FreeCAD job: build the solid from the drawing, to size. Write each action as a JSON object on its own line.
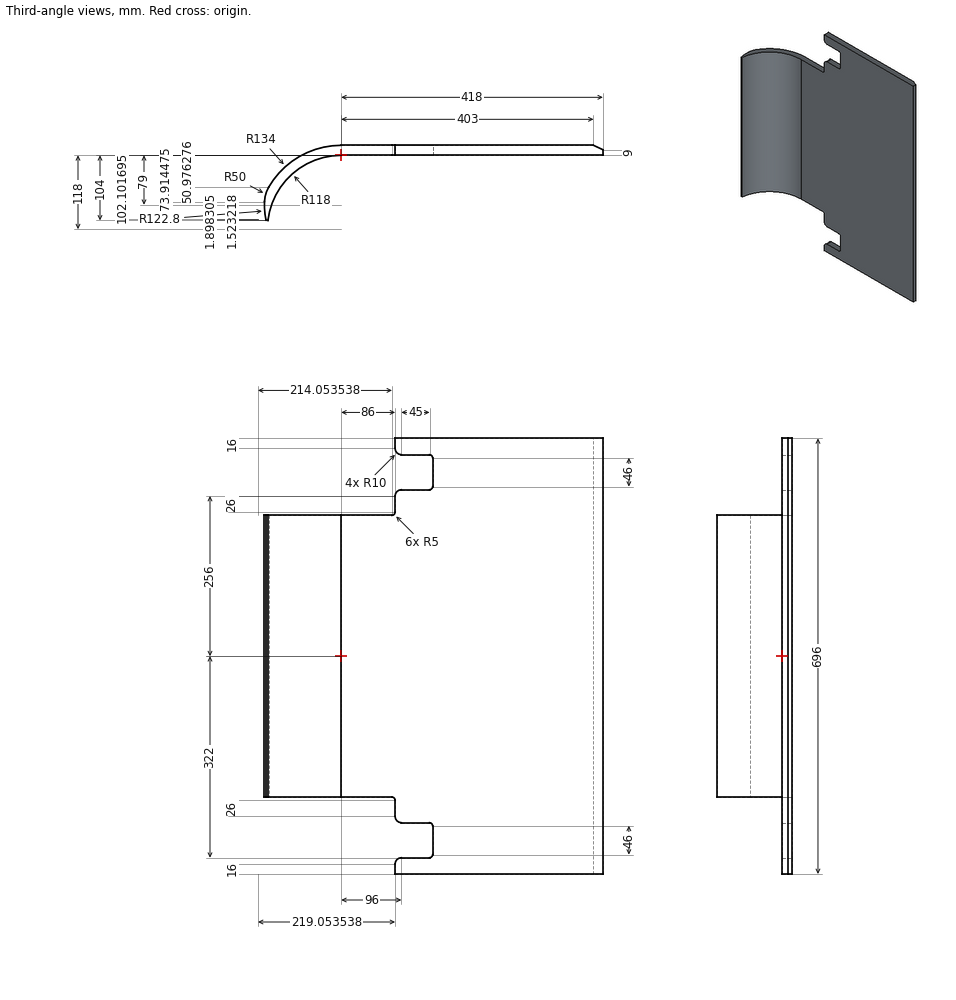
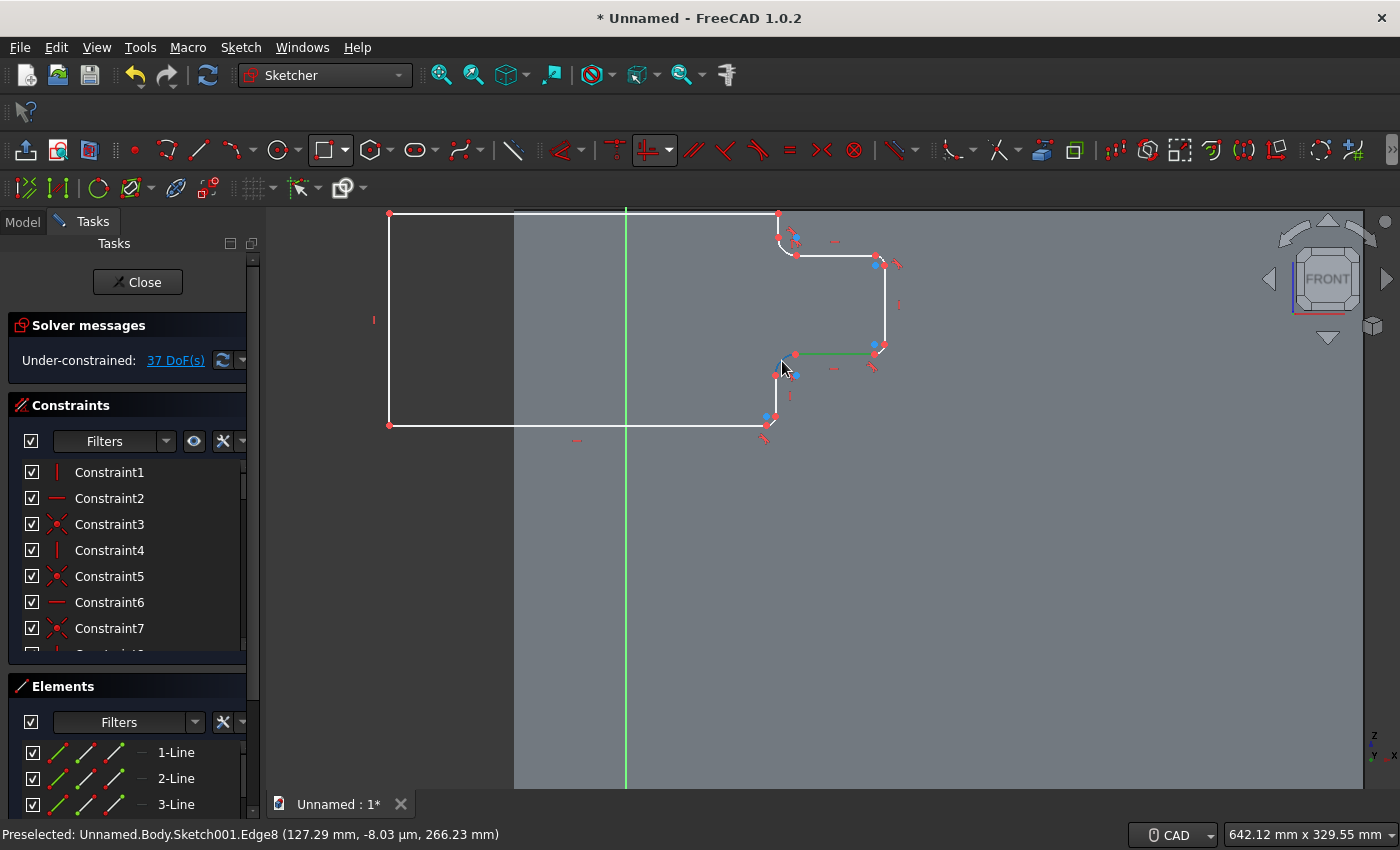
{"action": "left_click", "coordinate": [781, 361]}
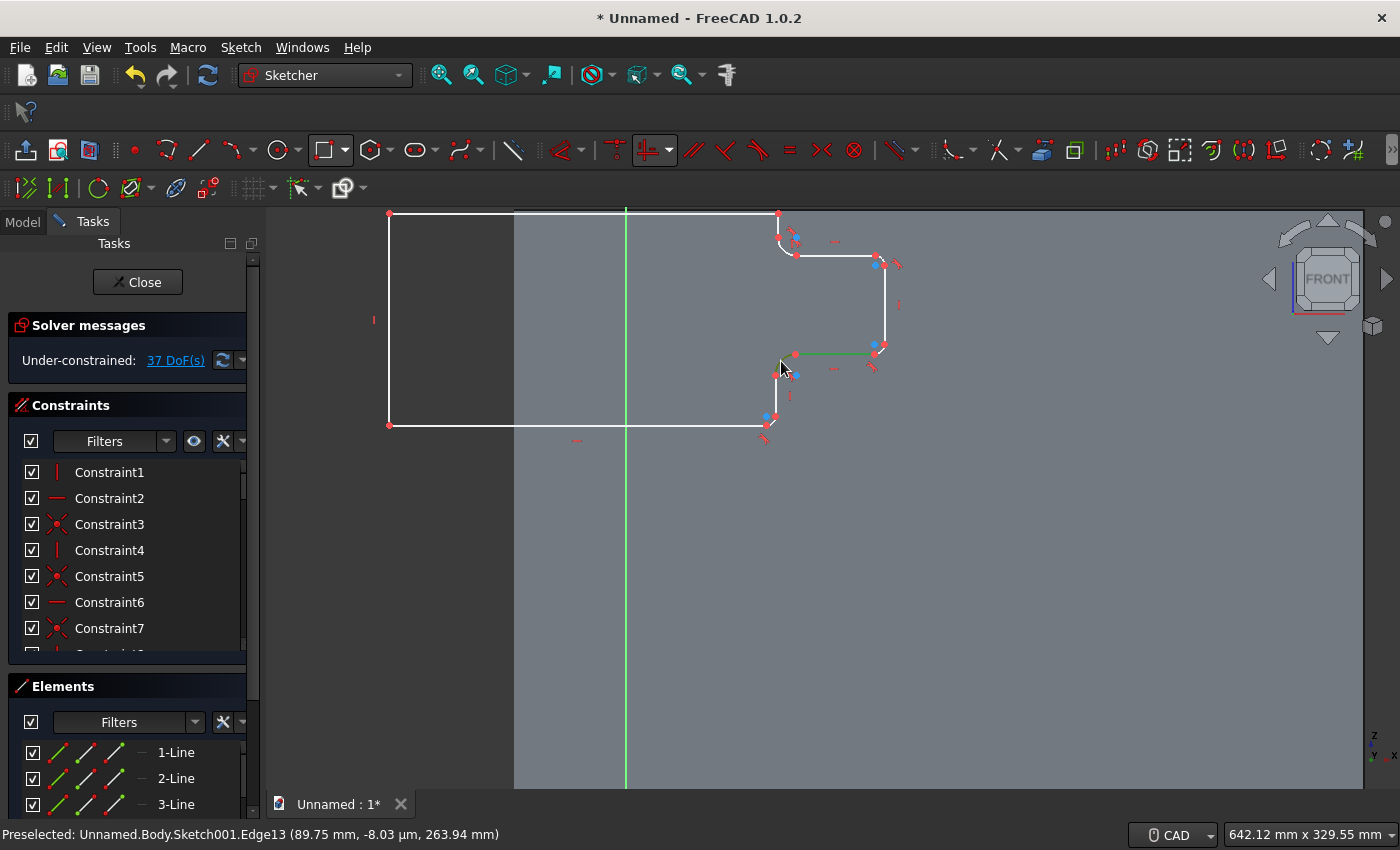
{"action": "left_click", "coordinate": [758, 150]}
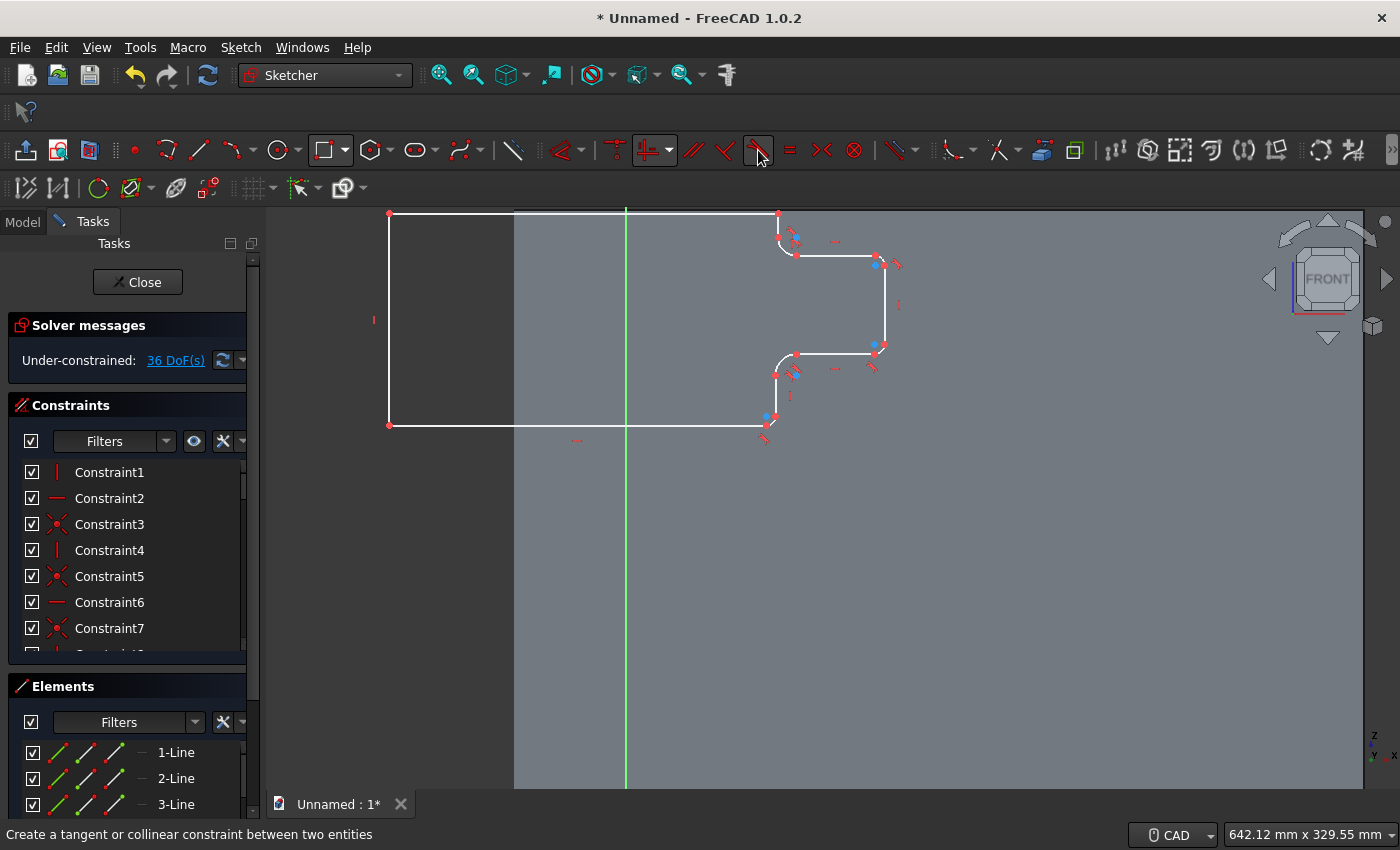
{"action": "scroll", "coordinate": [819, 357], "scroll_direction": "down", "scroll_amount": 6}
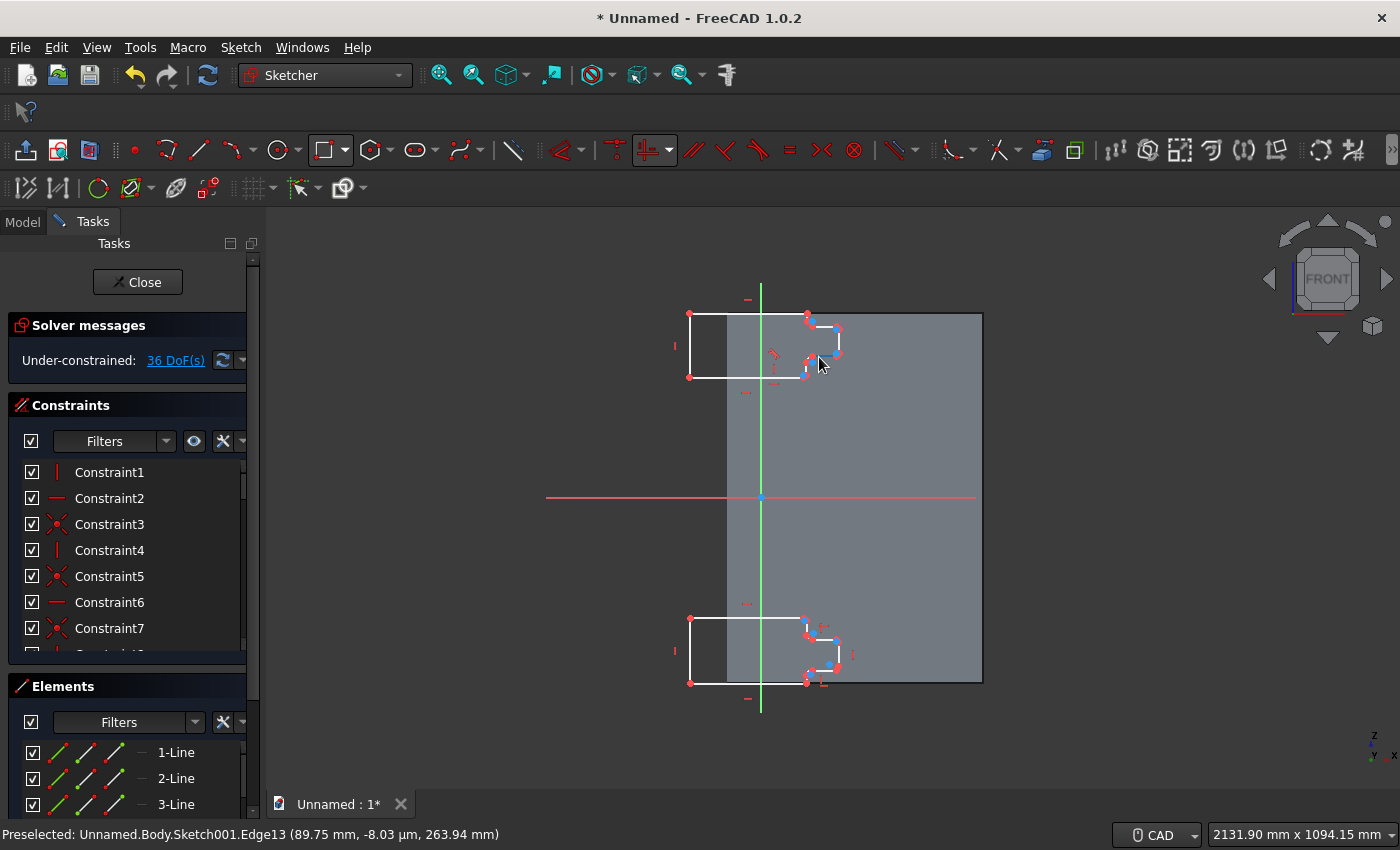
{"action": "scroll", "coordinate": [829, 671], "scroll_direction": "up", "scroll_amount": 4}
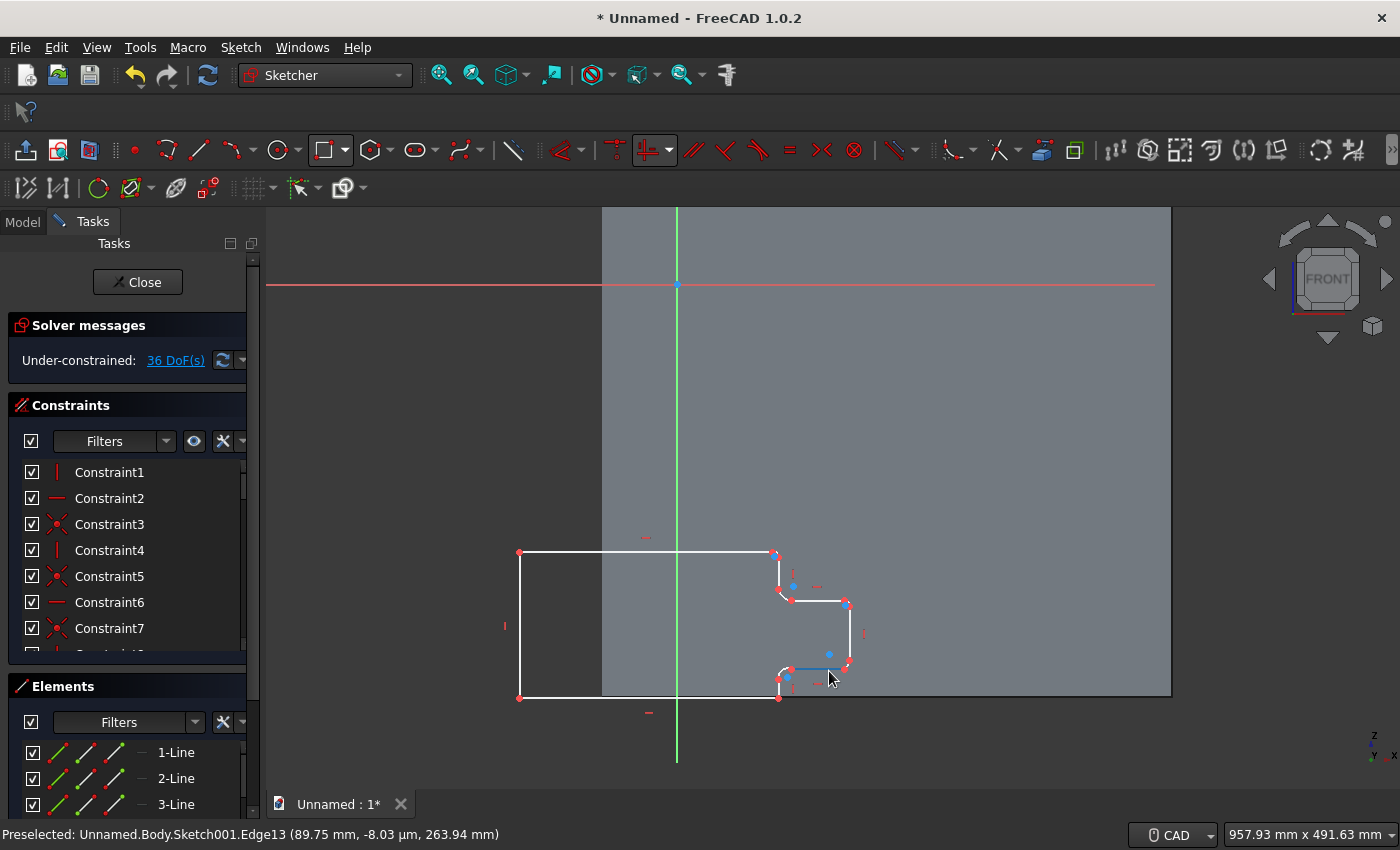
{"action": "left_click", "coordinate": [829, 669]}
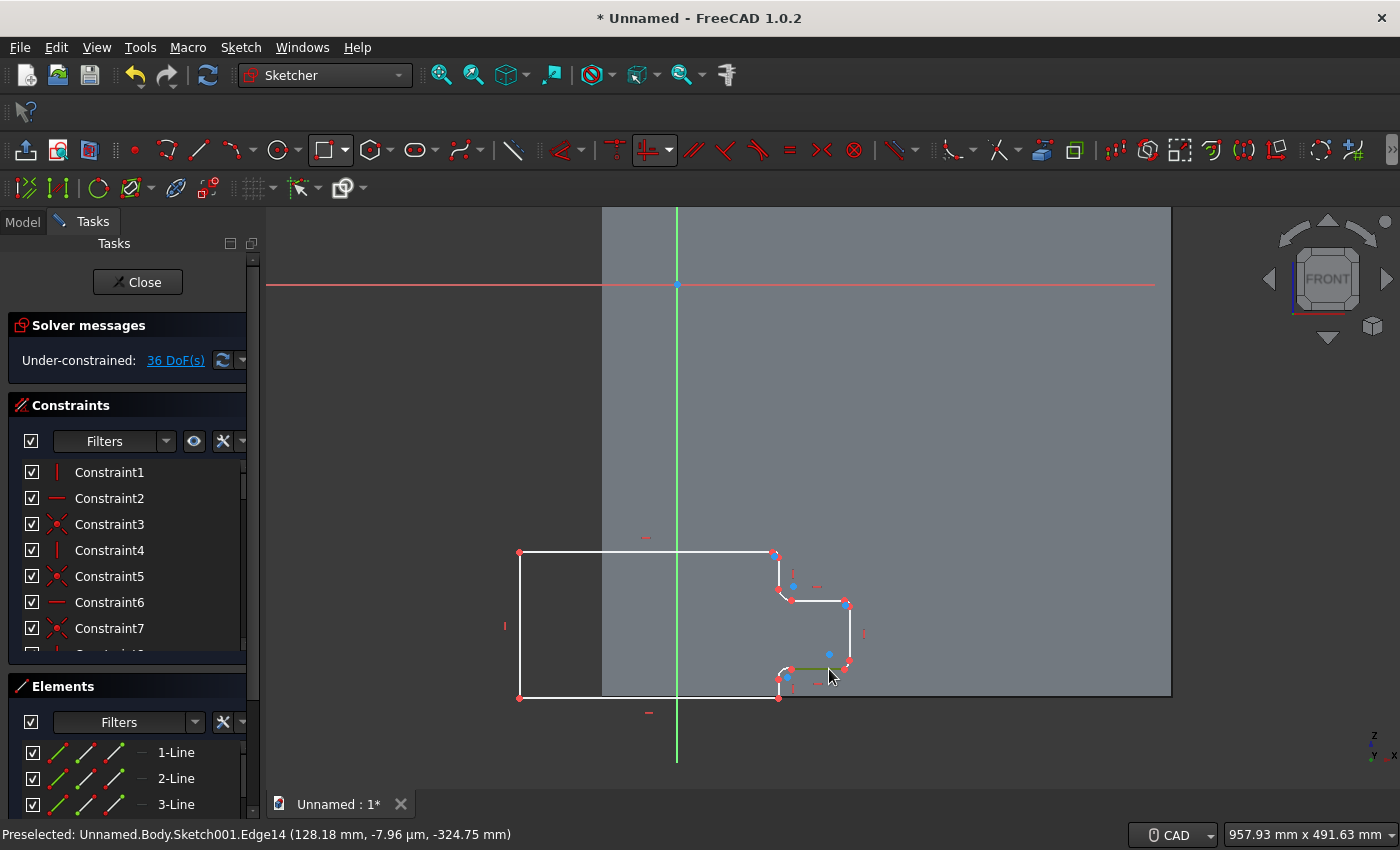
{"action": "scroll", "coordinate": [782, 670], "scroll_direction": "up", "scroll_amount": 3}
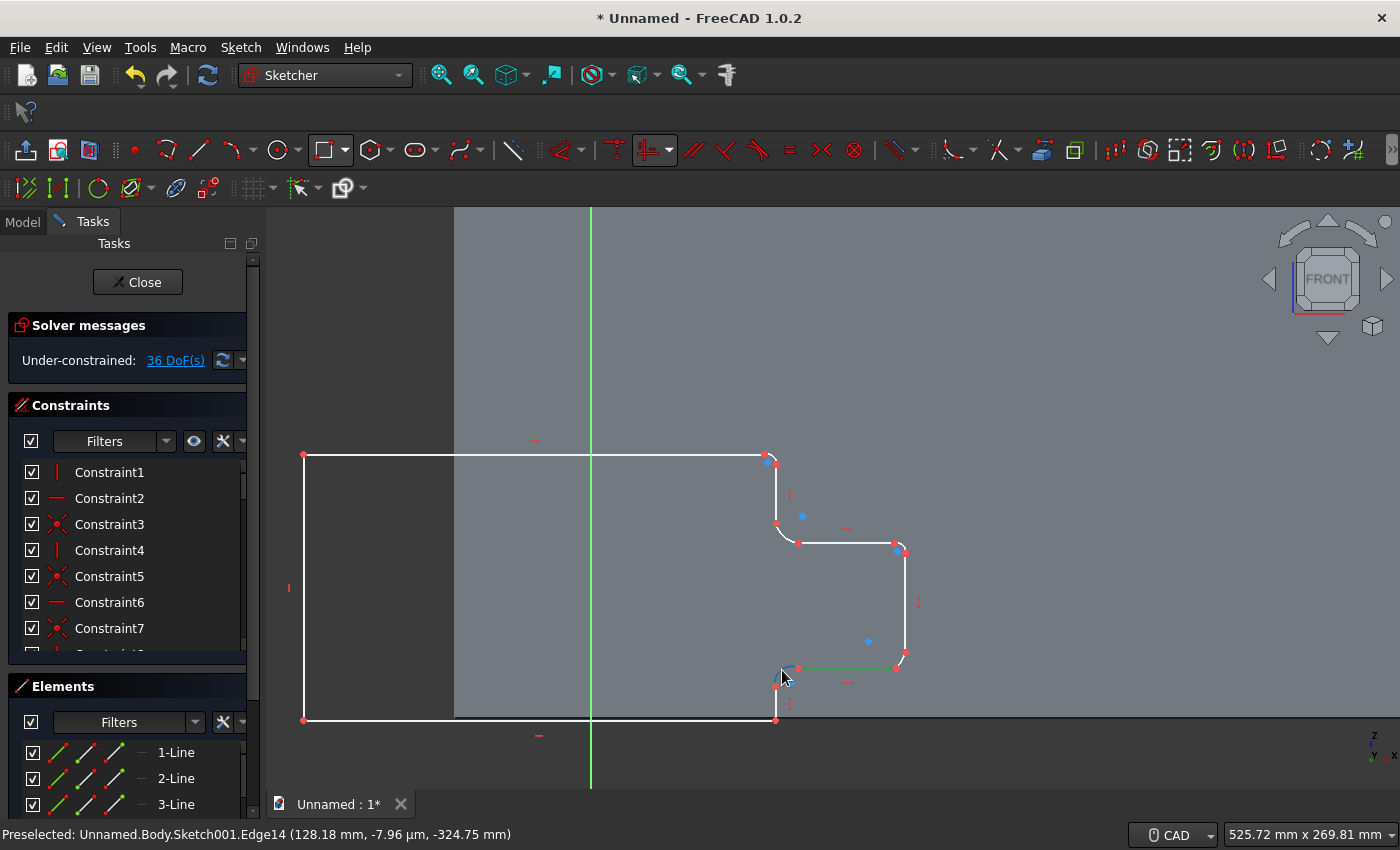
{"action": "left_click", "coordinate": [781, 670]}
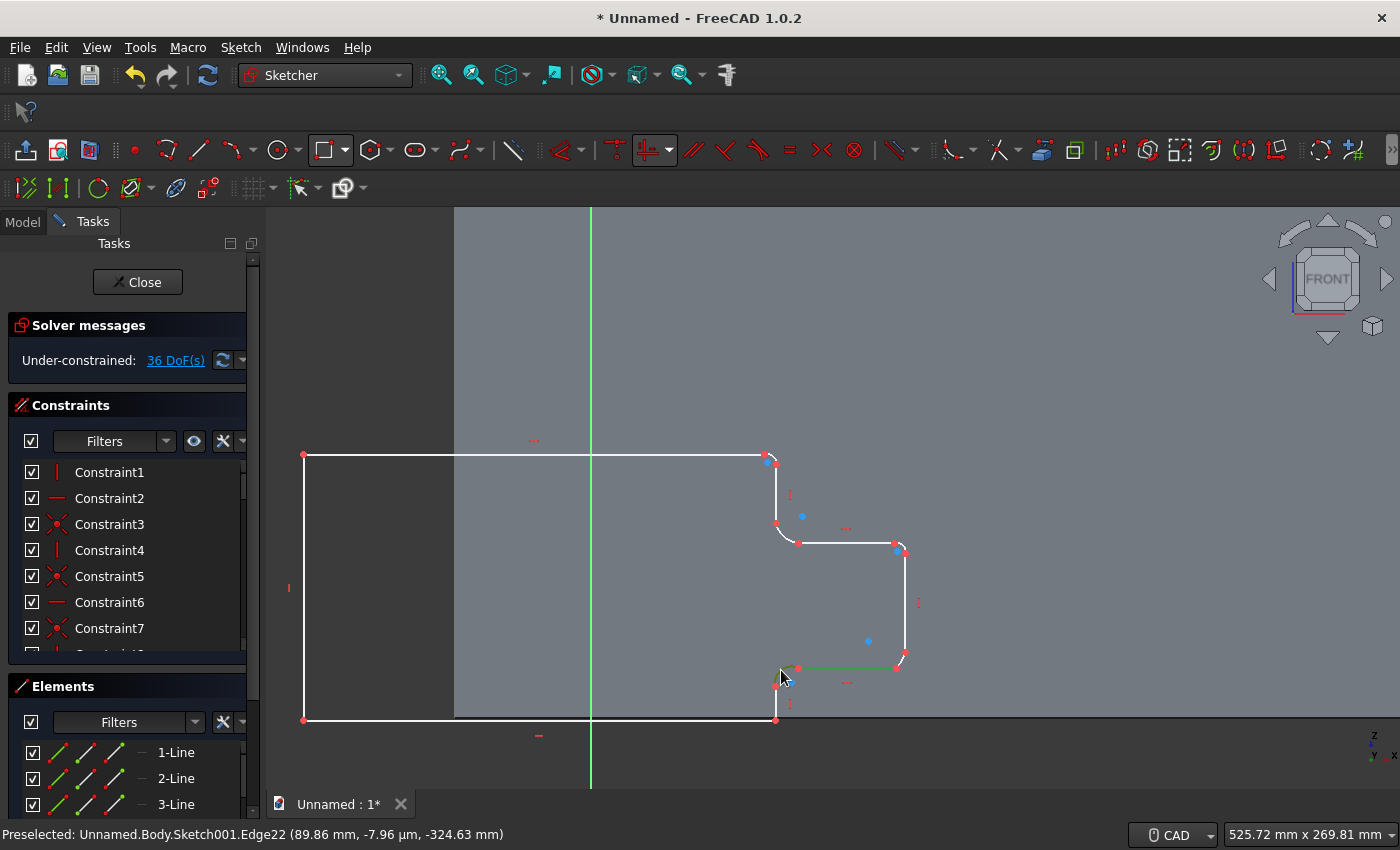
{"action": "left_click", "coordinate": [758, 150]}